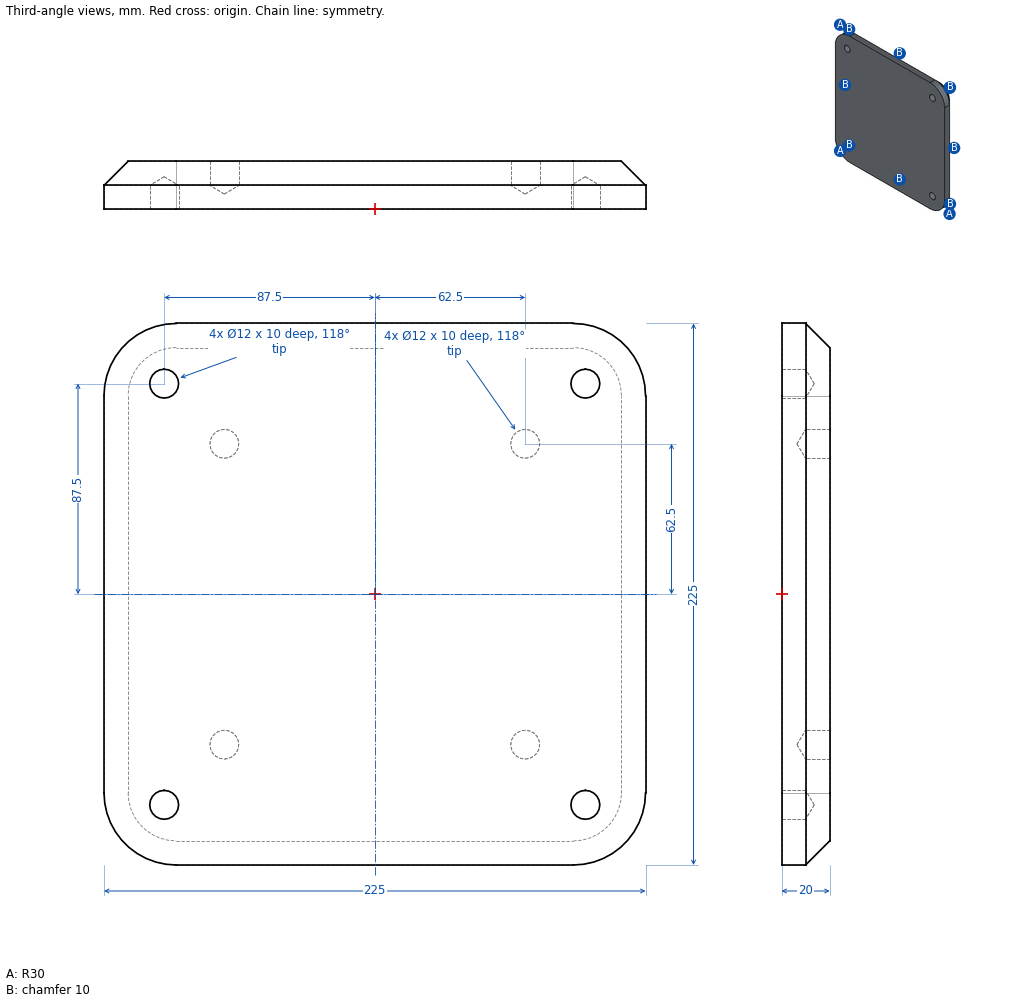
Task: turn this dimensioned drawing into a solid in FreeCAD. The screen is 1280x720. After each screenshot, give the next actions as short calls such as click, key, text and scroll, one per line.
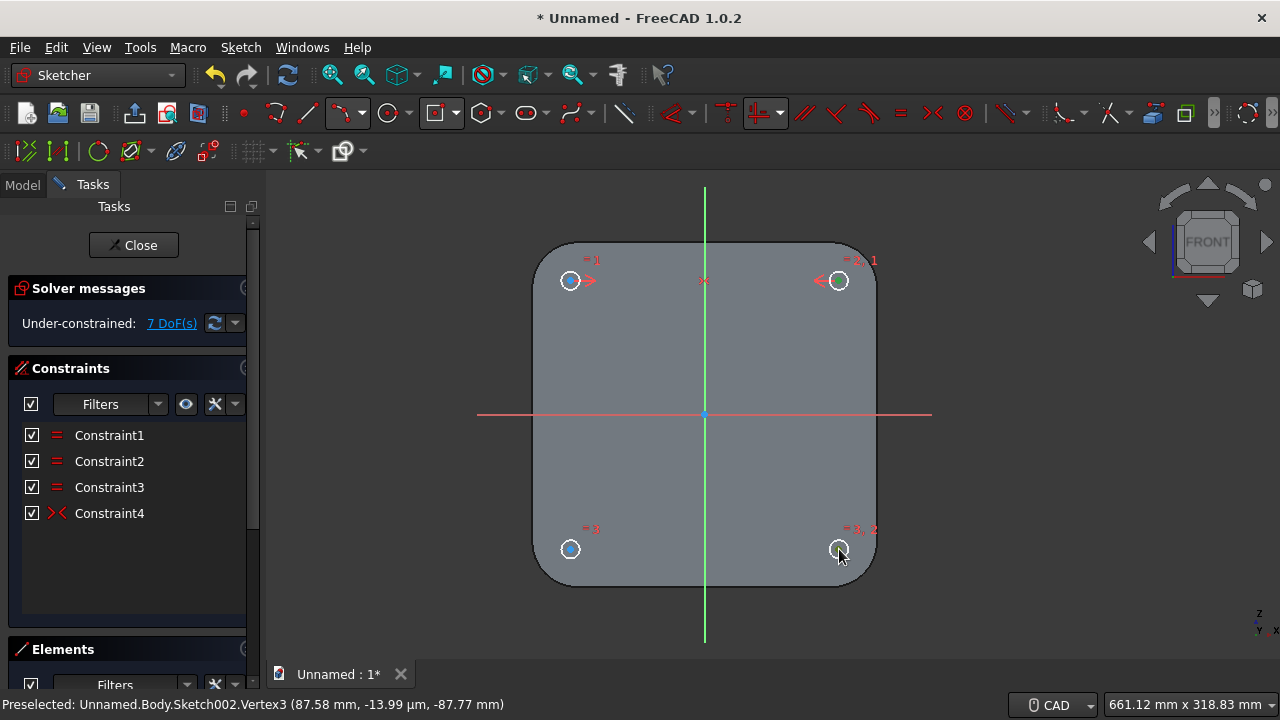
click(529, 415)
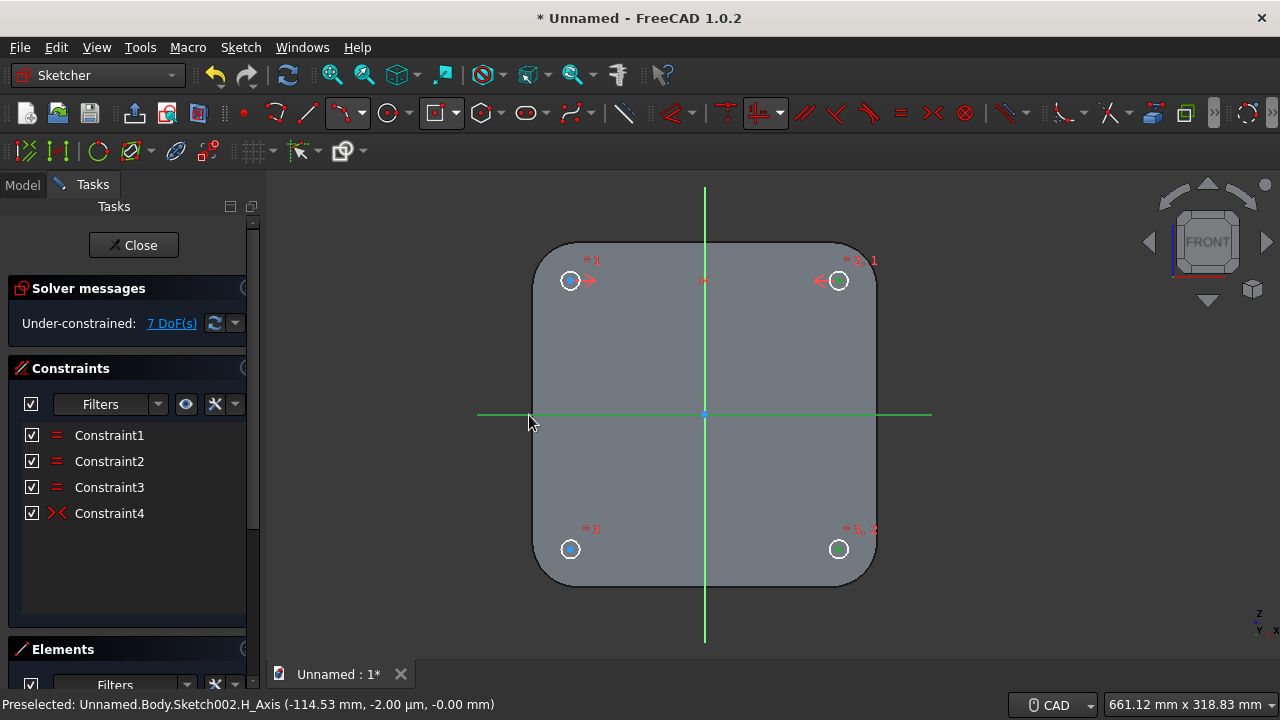
click(934, 114)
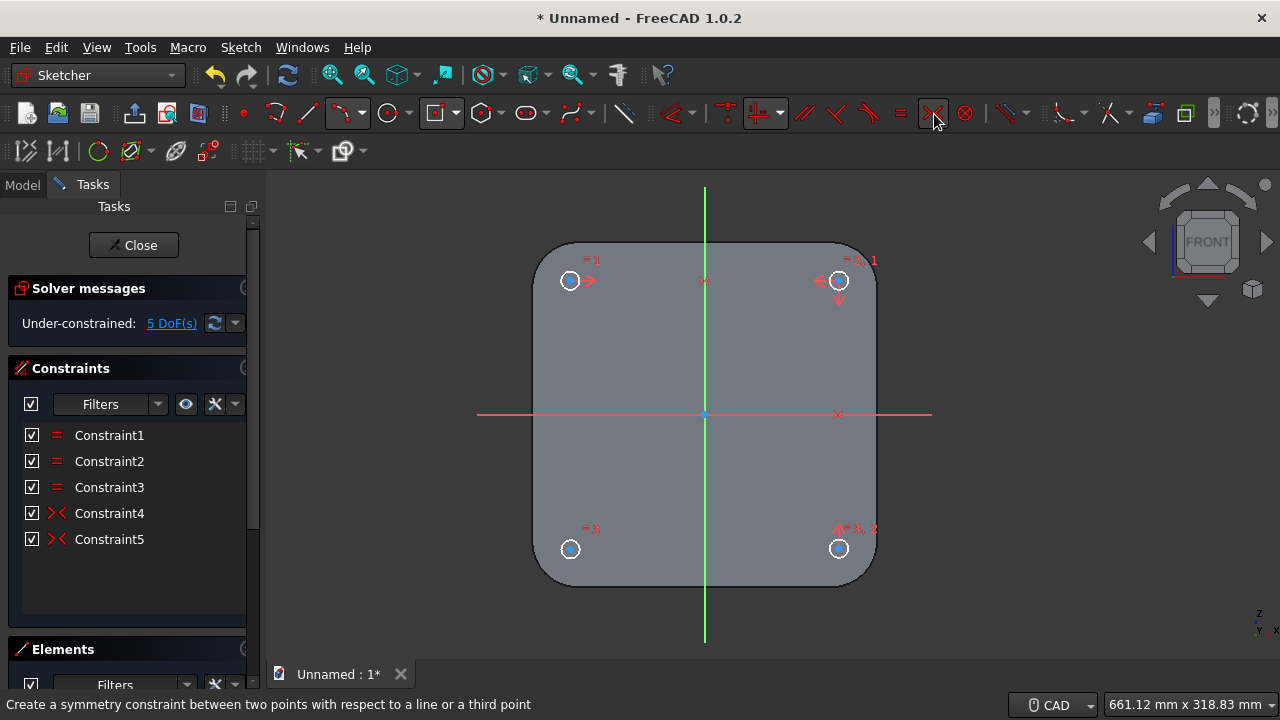
click(570, 281)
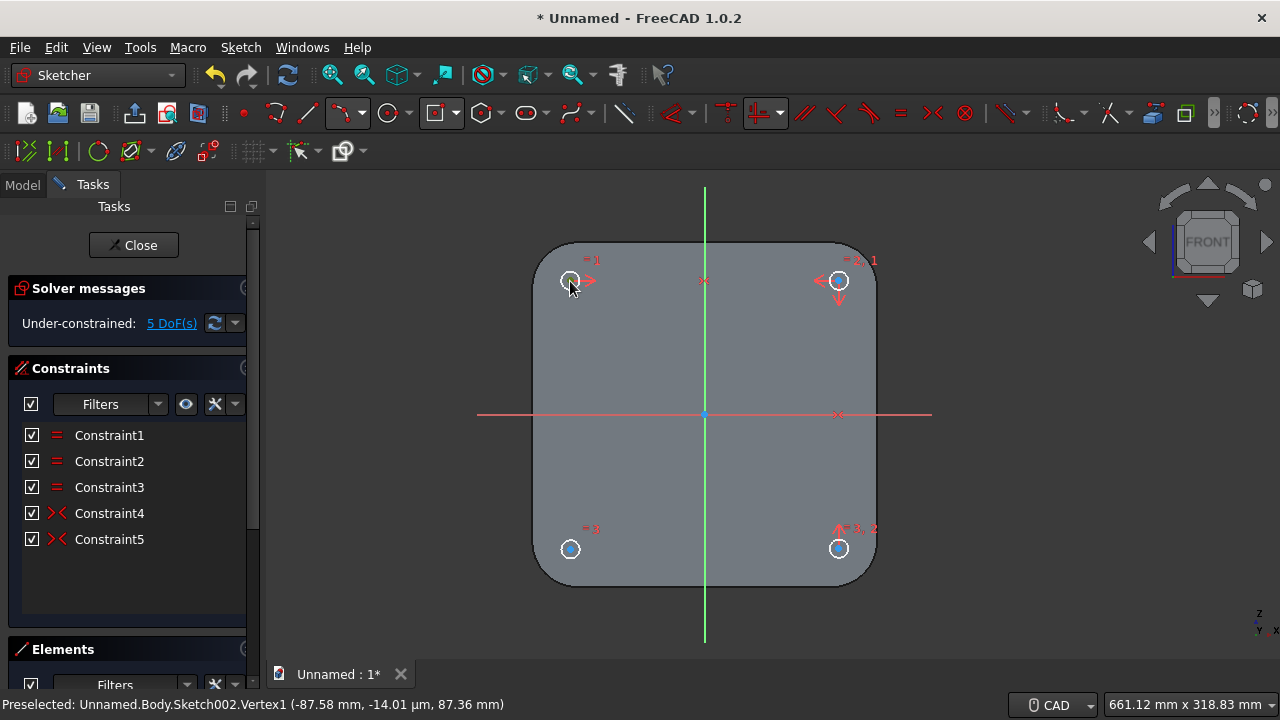
click(571, 549)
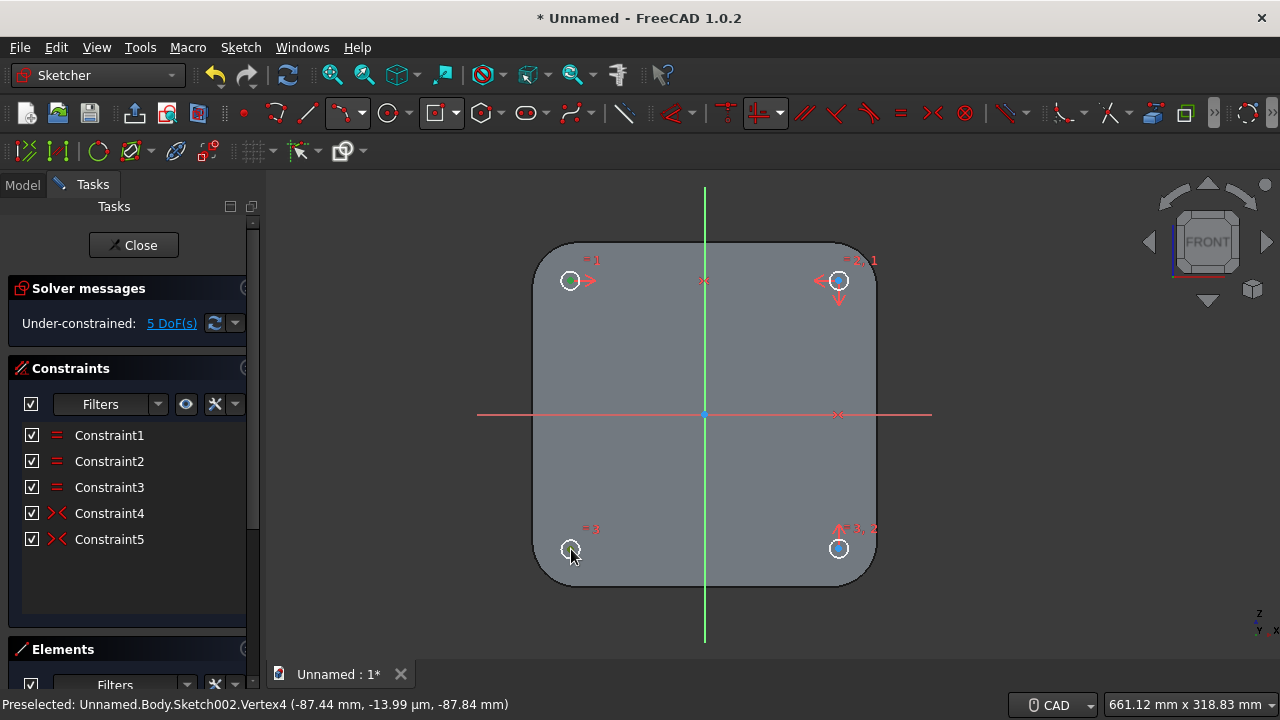
click(529, 415)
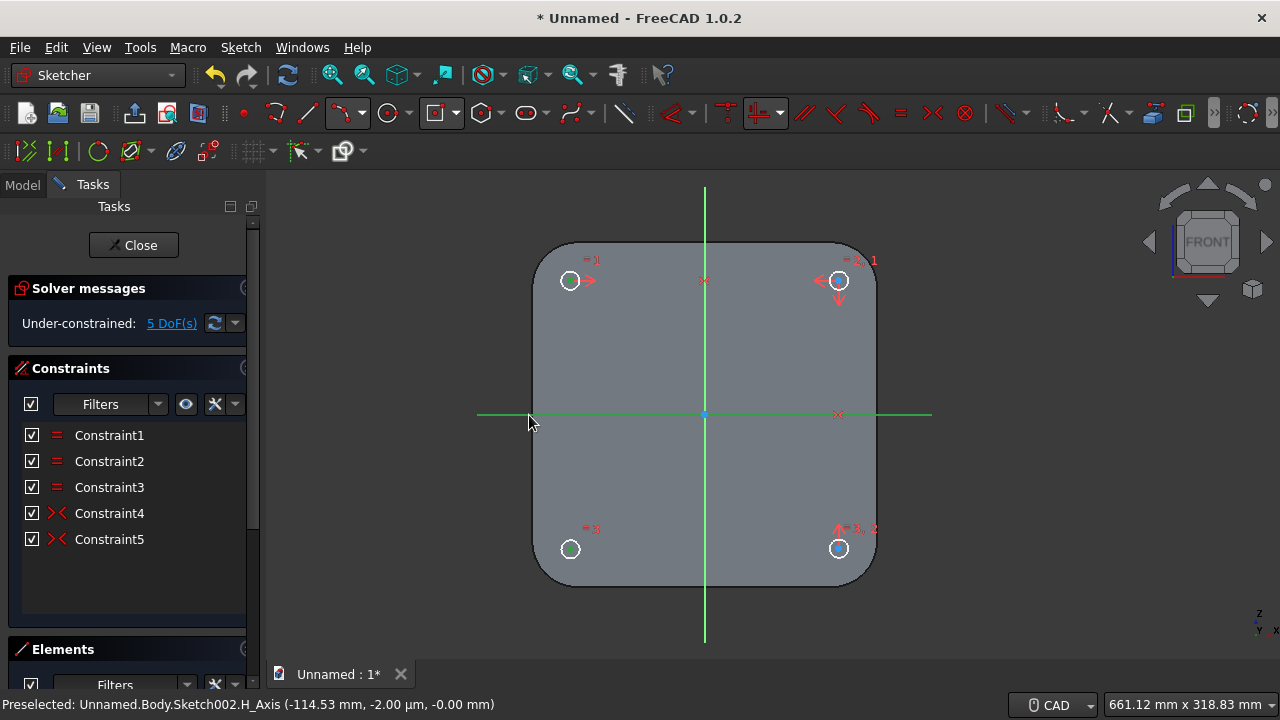
click(934, 114)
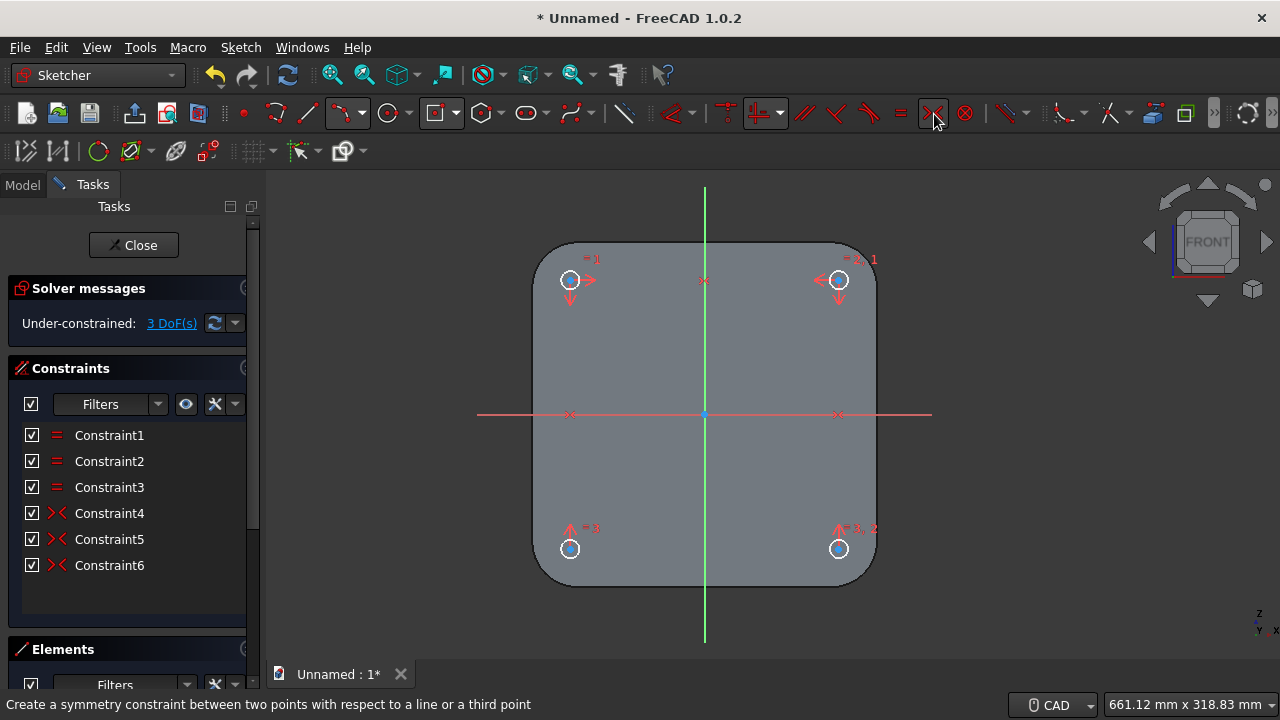
click(672, 114)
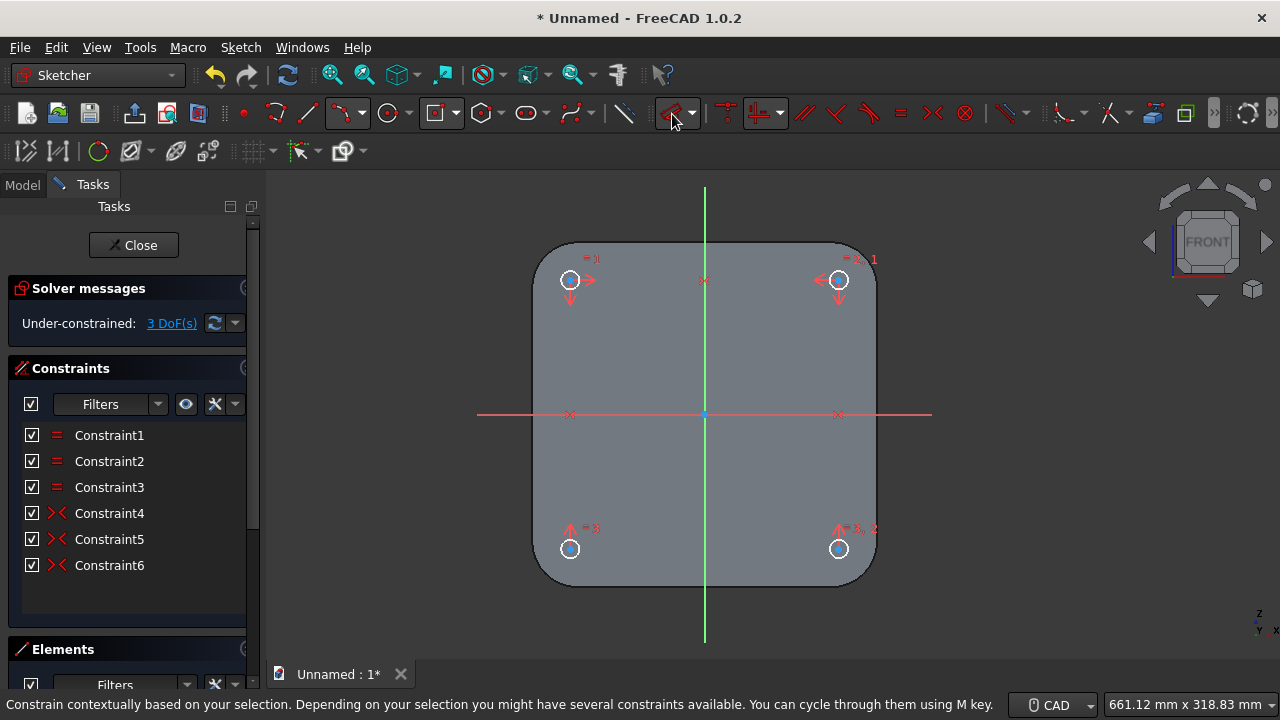
scroll(577, 274, up, 4)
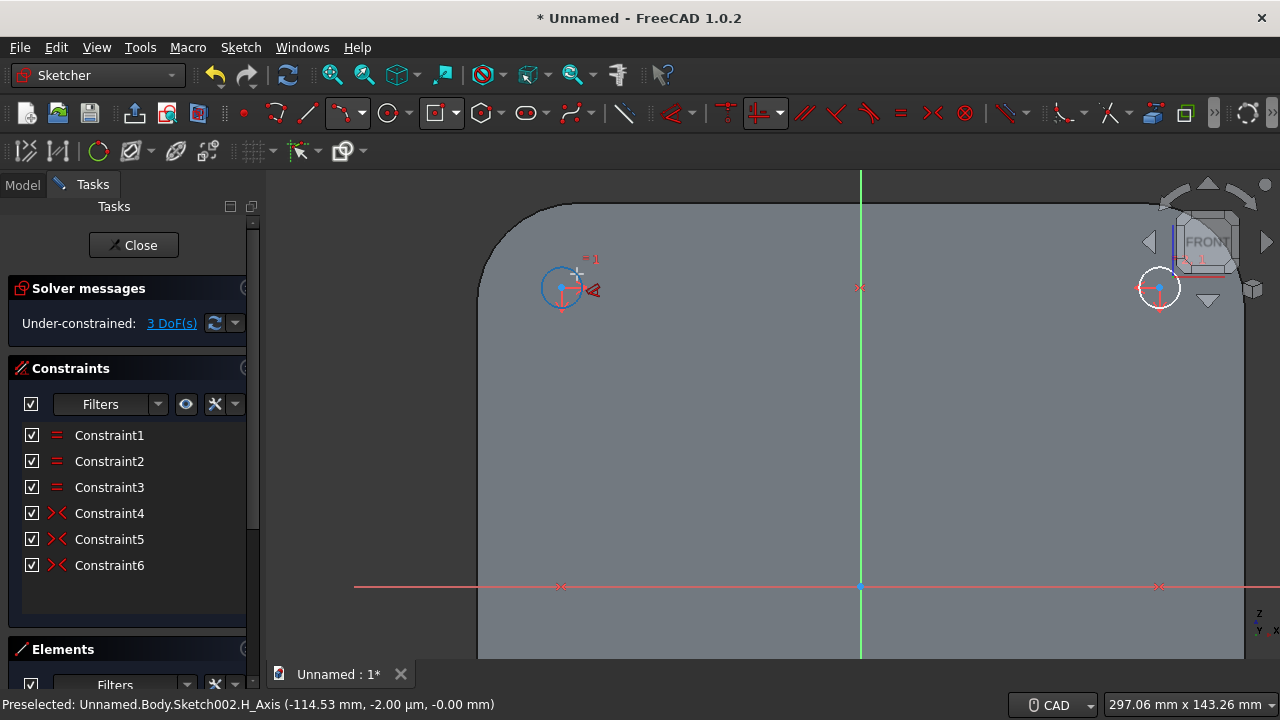
click(576, 273)
click(598, 250)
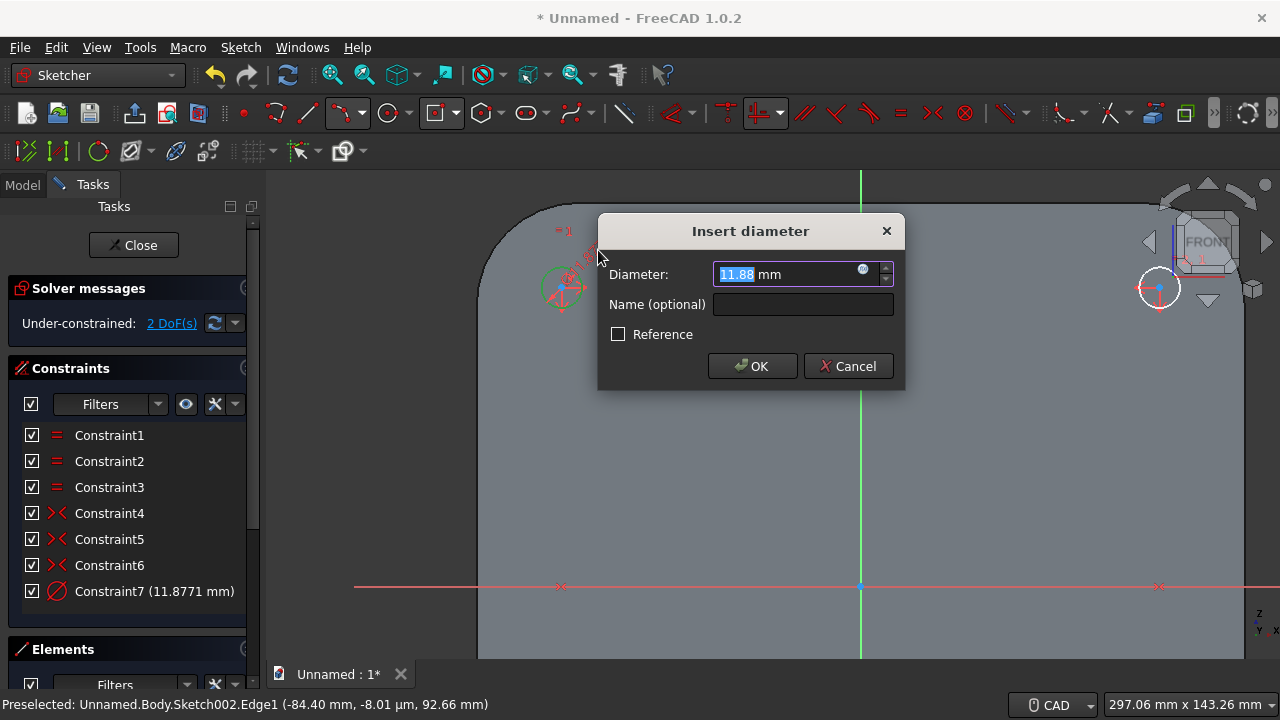
text(12)
key(Return)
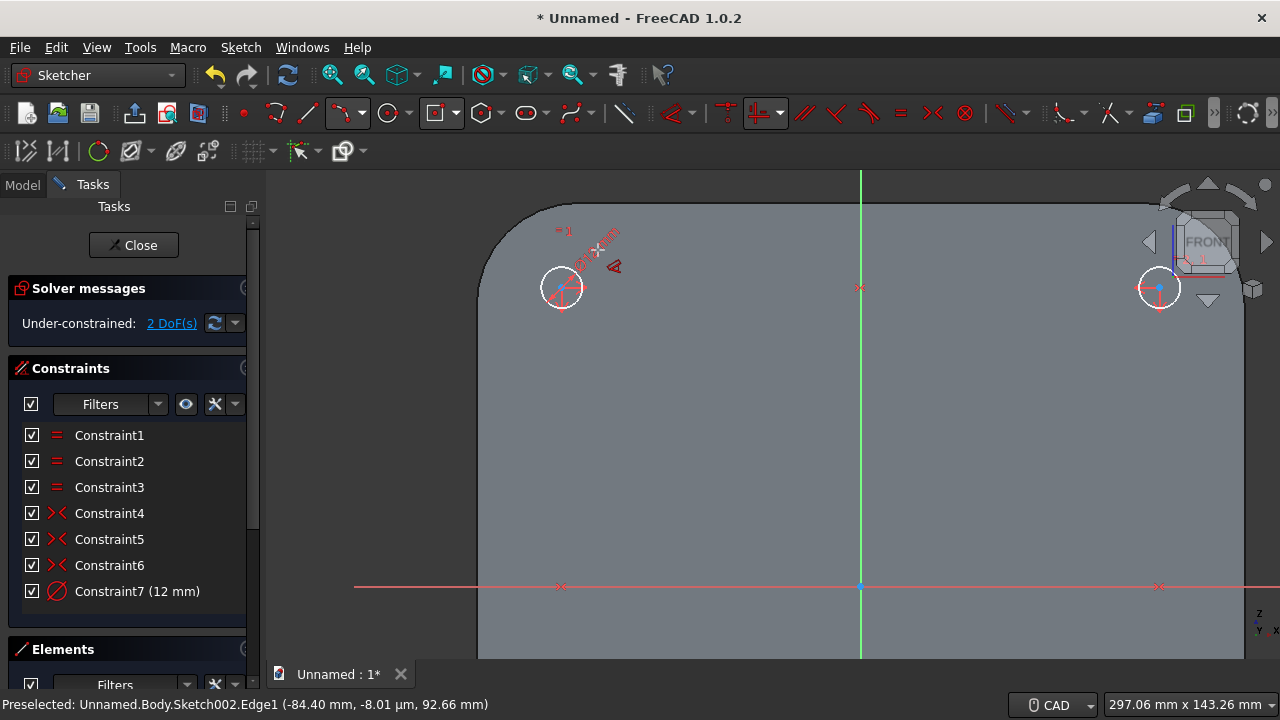
click(562, 288)
click(711, 254)